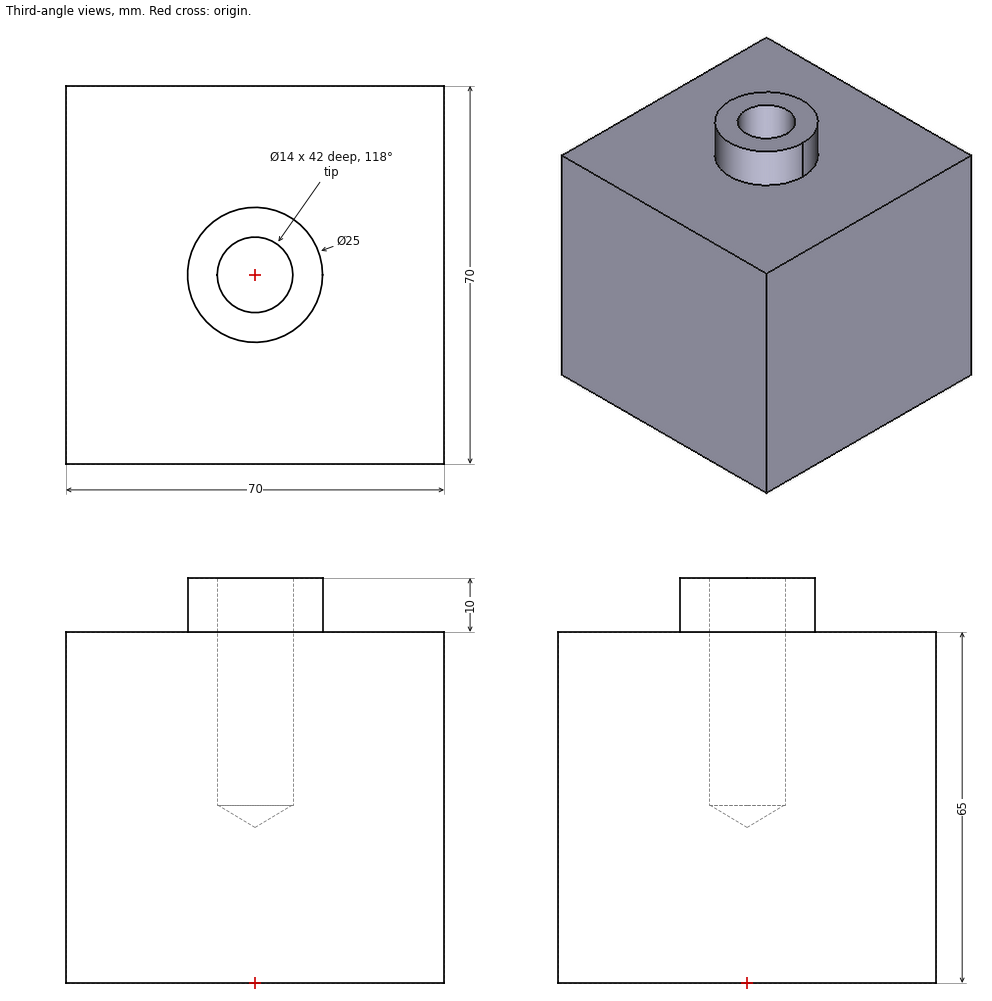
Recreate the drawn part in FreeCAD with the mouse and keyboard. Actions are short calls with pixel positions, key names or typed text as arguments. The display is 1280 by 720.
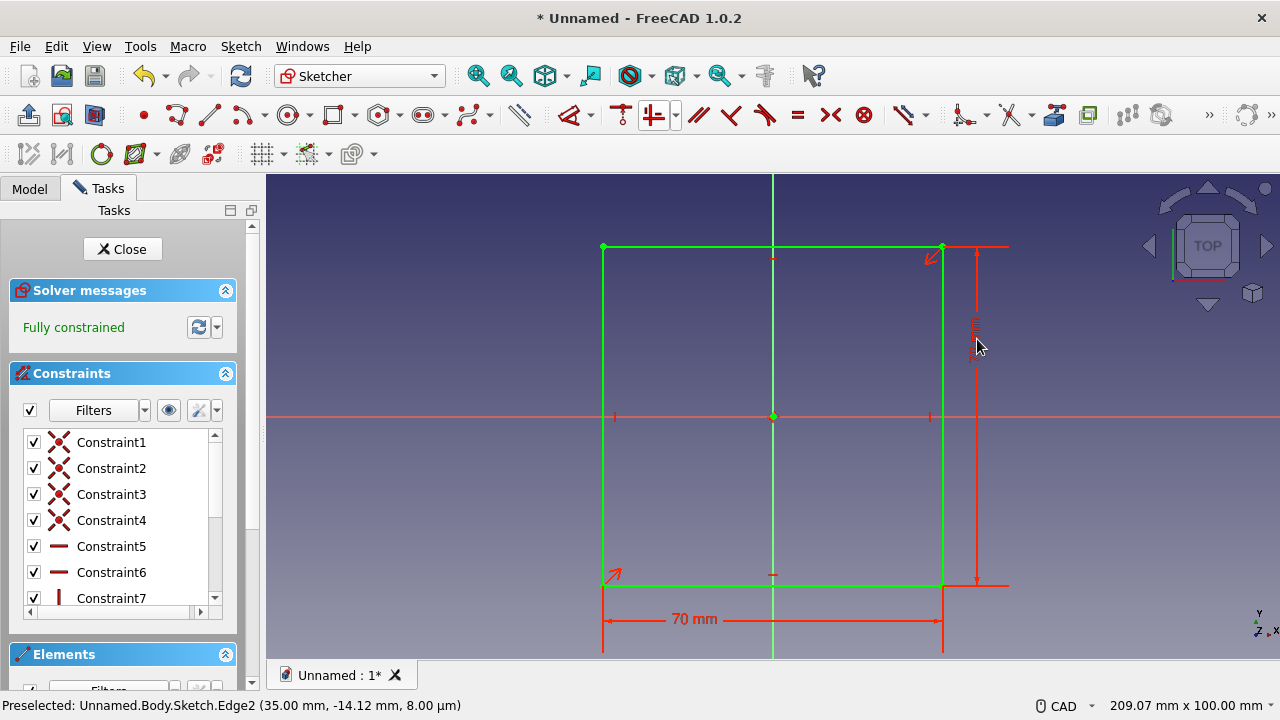
click(123, 249)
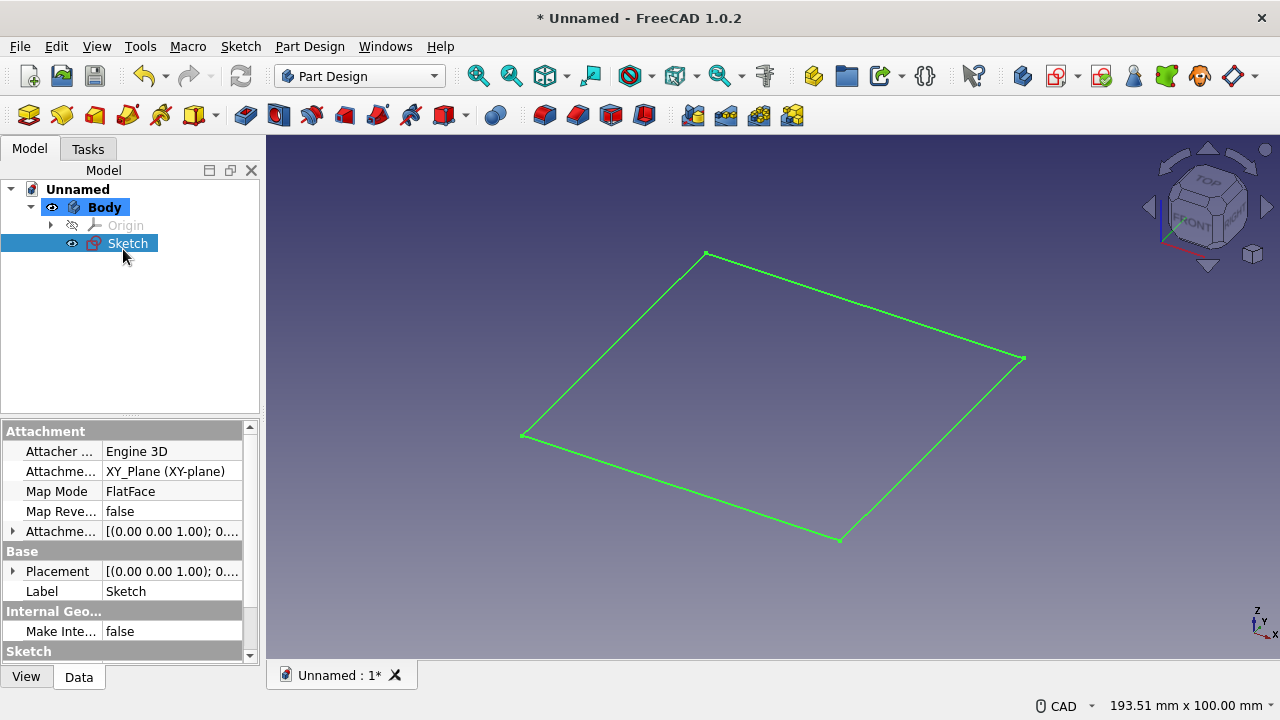
click(29, 116)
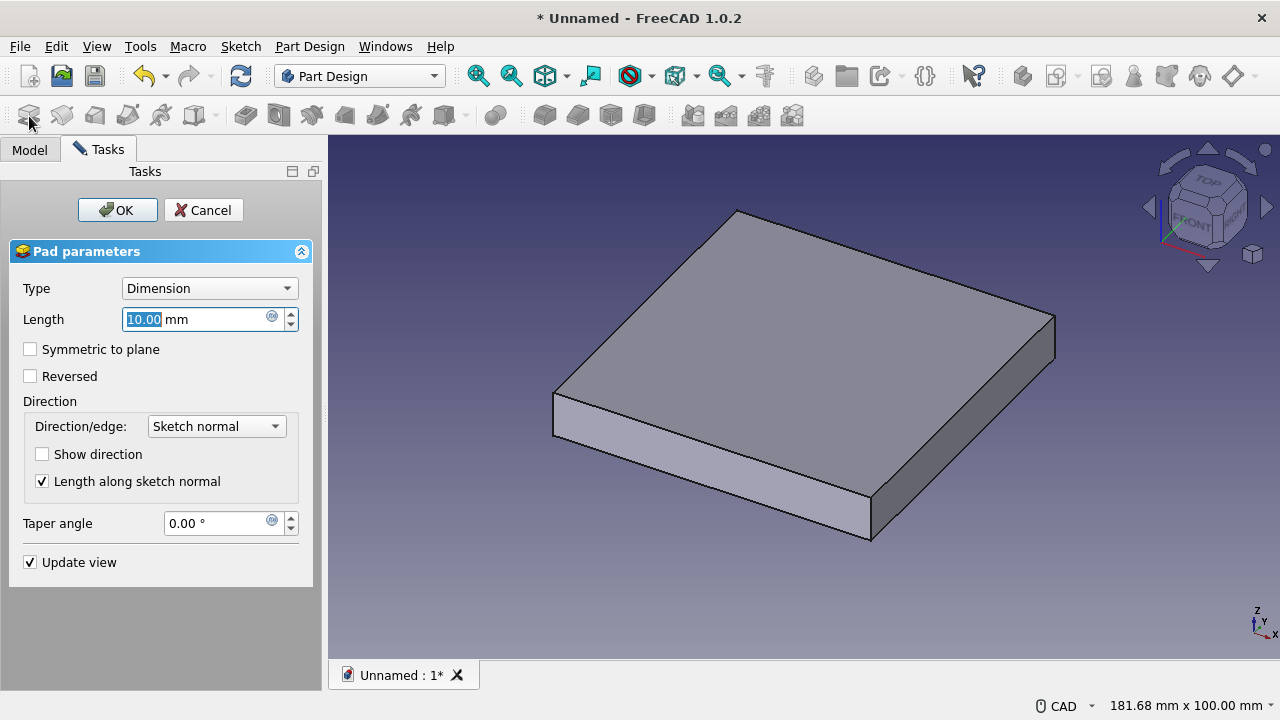
text(65)
key(Tab)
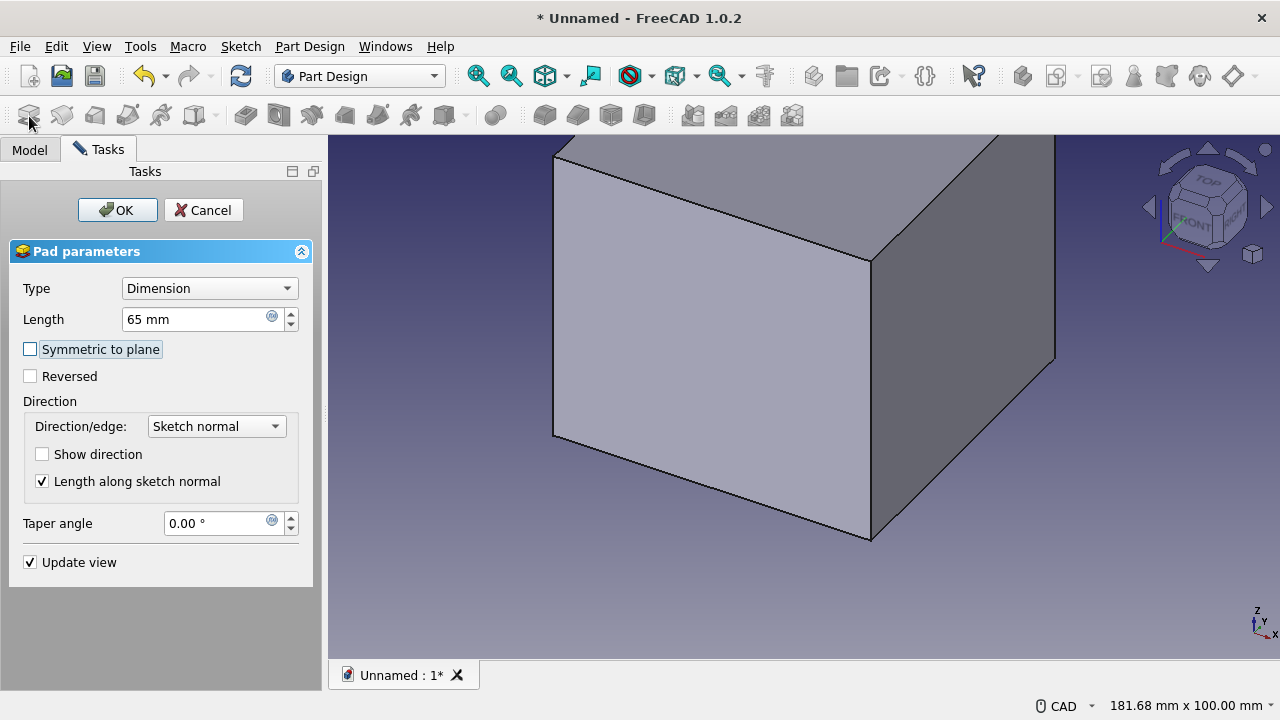
click(118, 210)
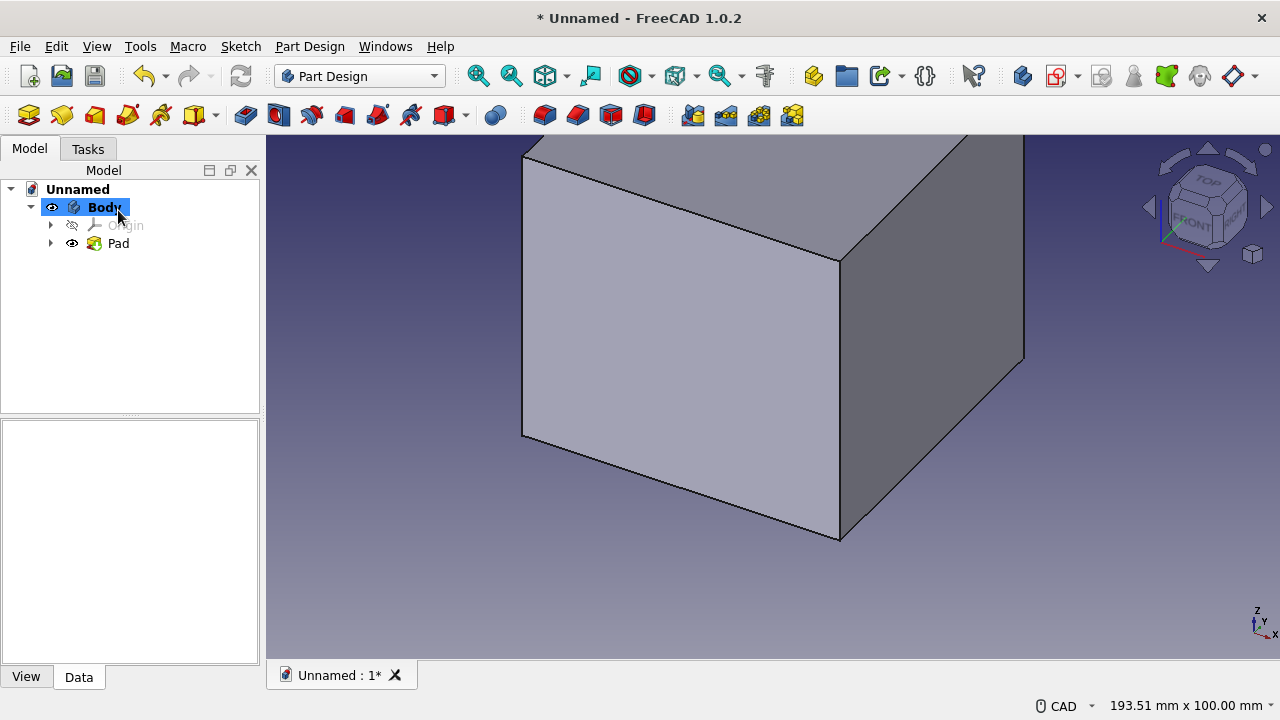
click(479, 76)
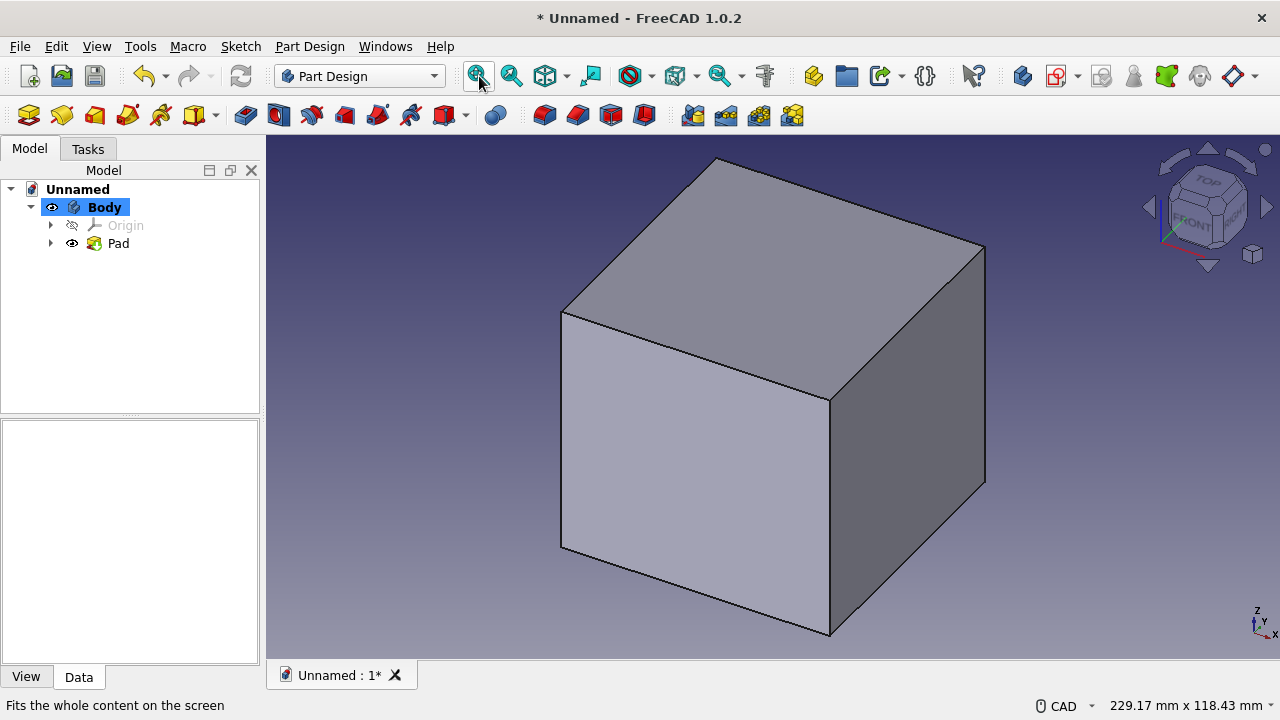
click(773, 278)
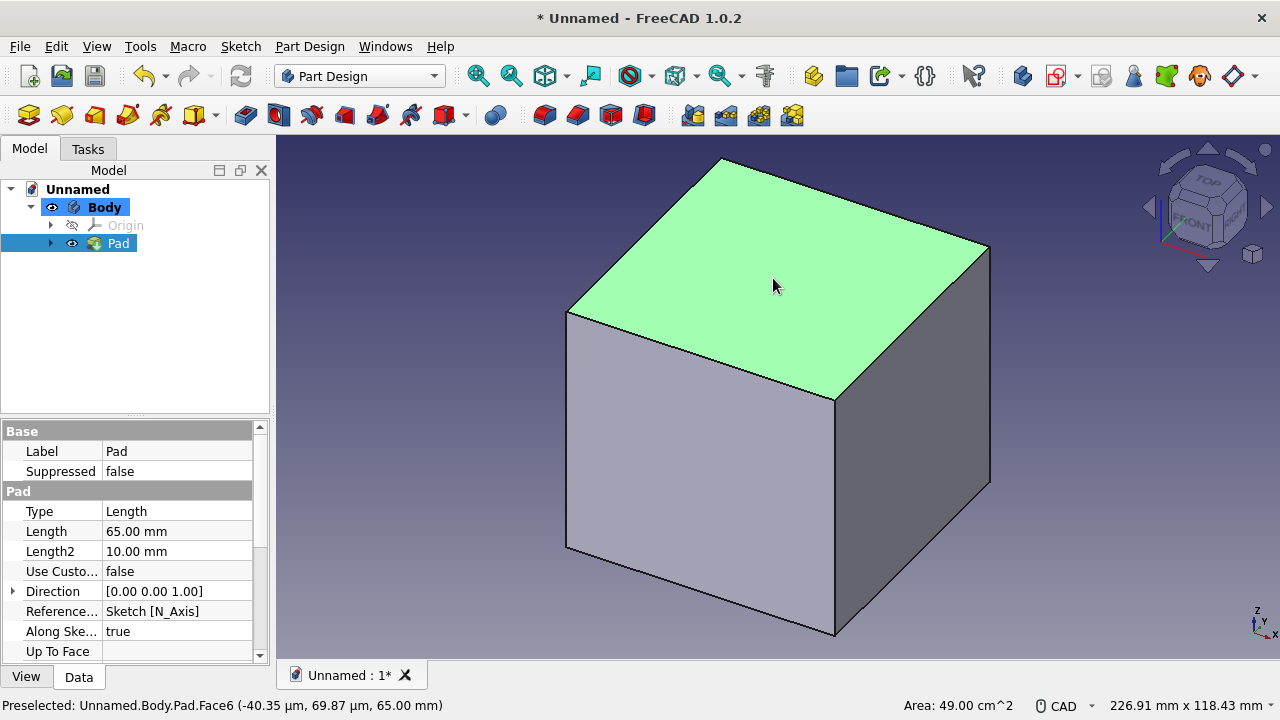
click(1056, 76)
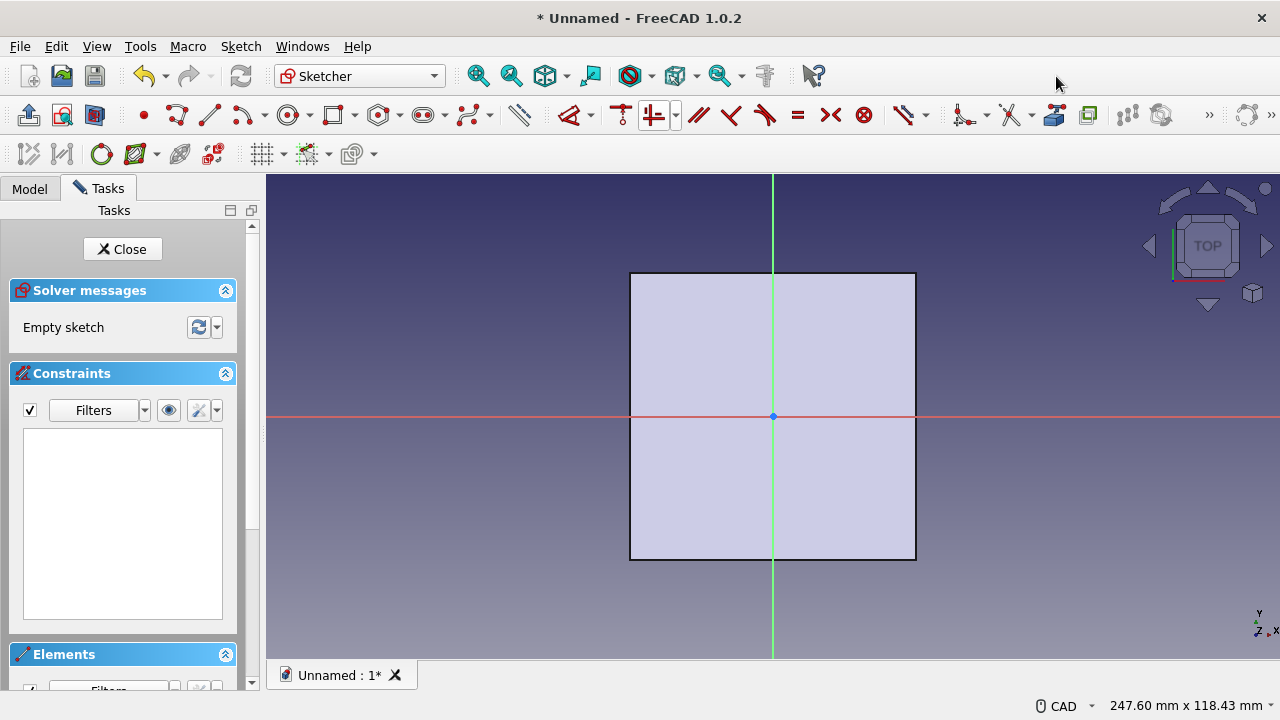
scroll(813, 416, up, 5)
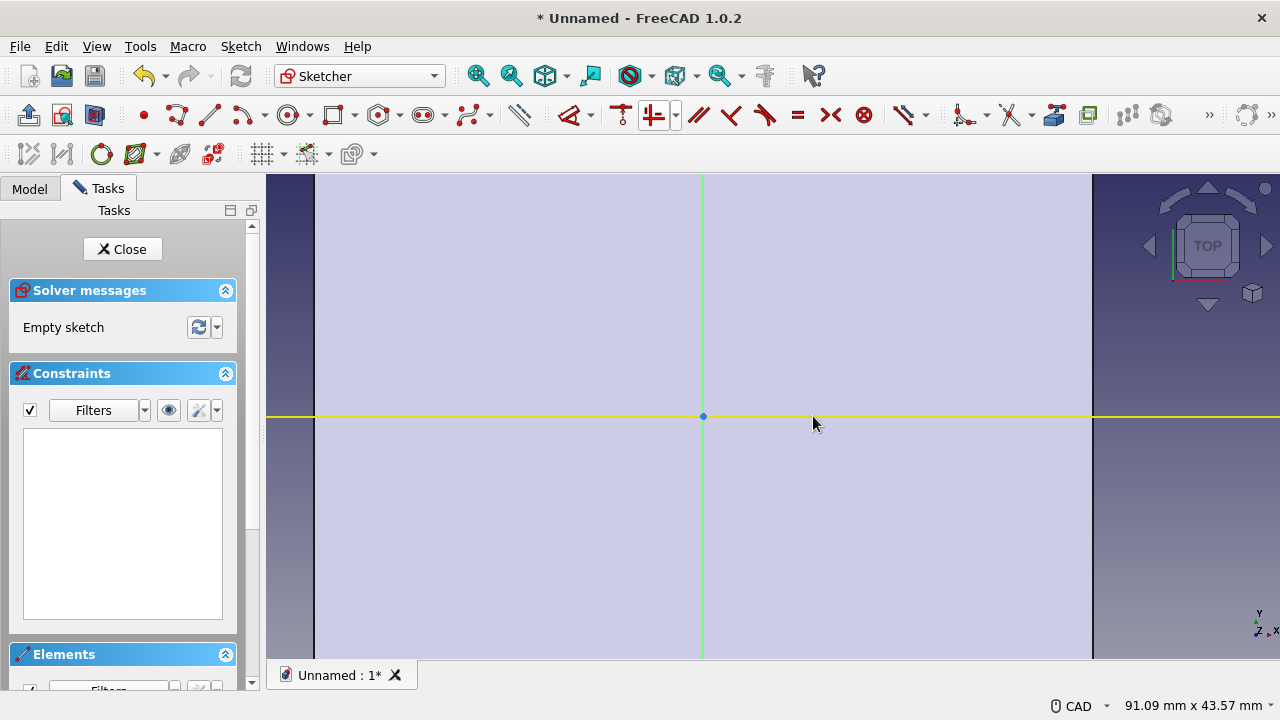
click(288, 116)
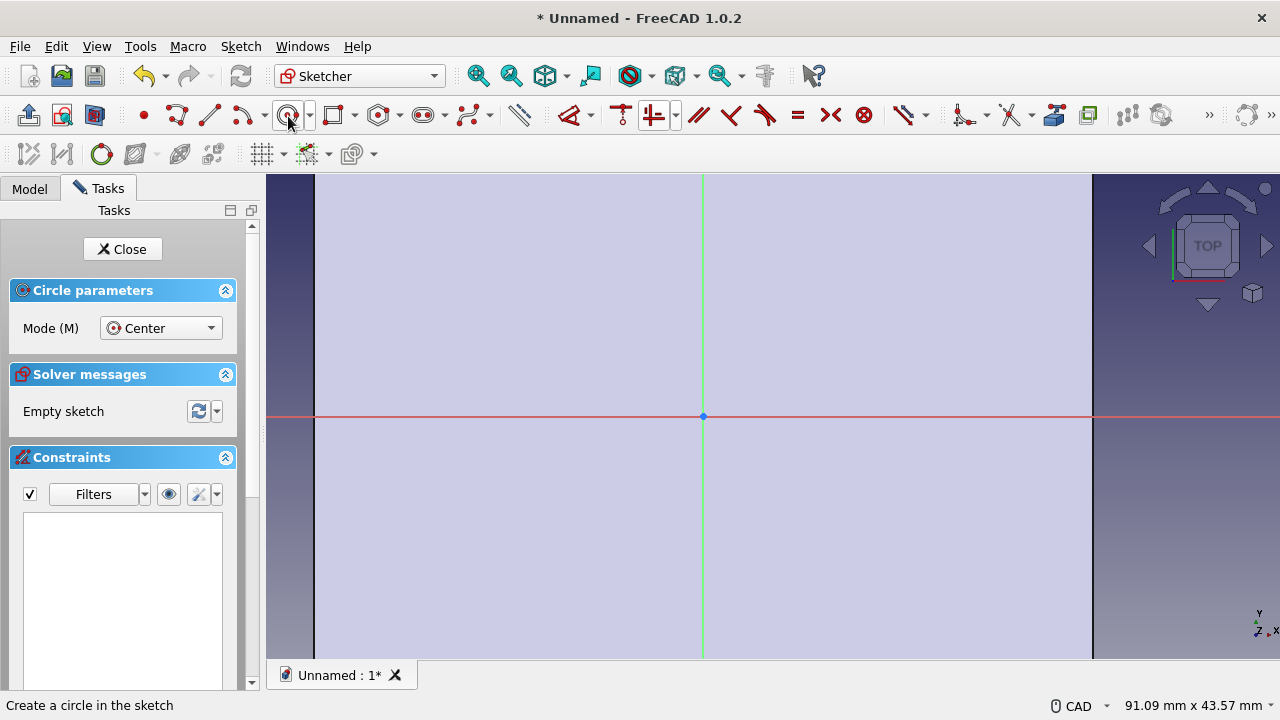
click(703, 416)
click(802, 318)
key(Escape)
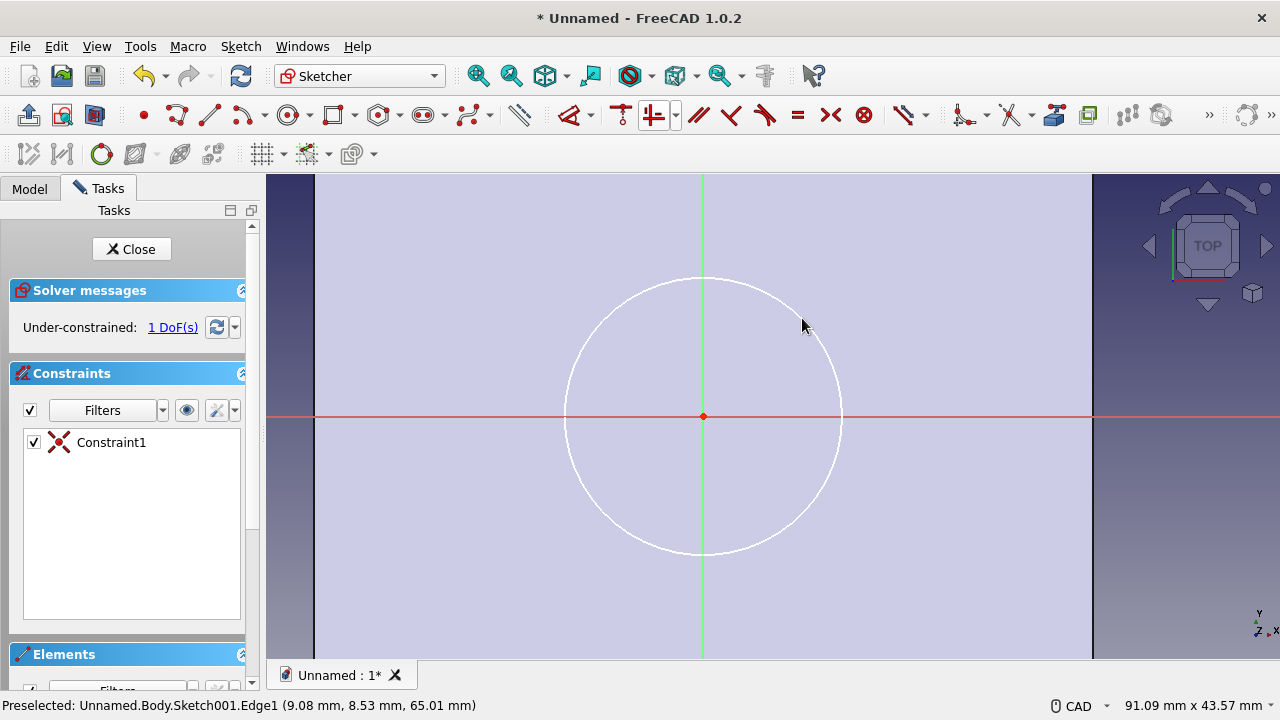
click(568, 116)